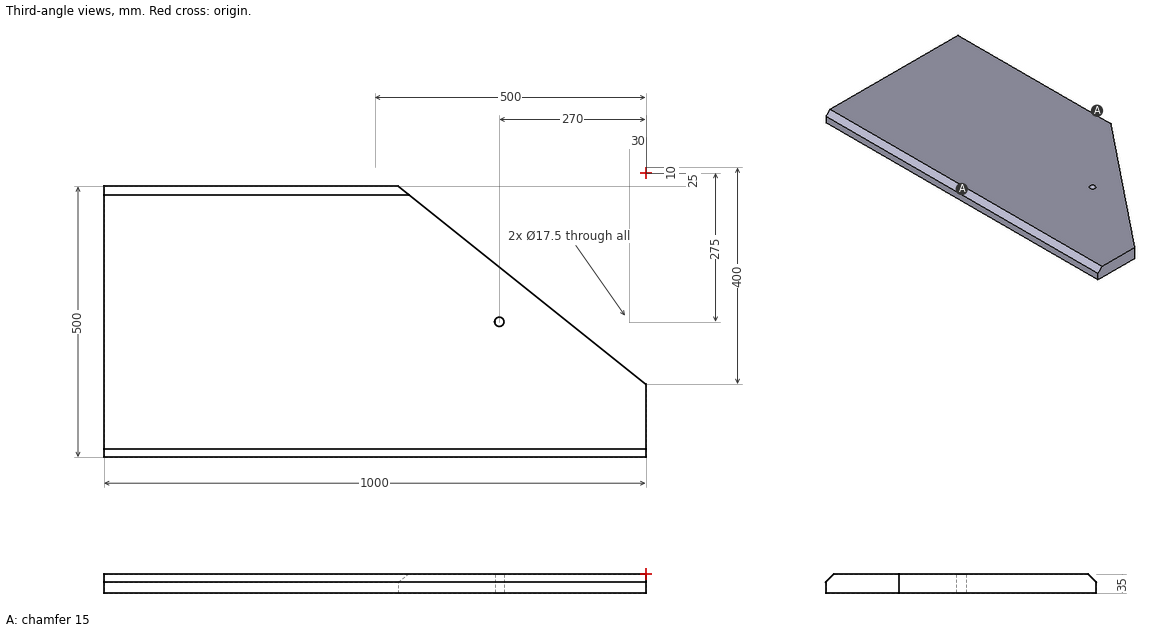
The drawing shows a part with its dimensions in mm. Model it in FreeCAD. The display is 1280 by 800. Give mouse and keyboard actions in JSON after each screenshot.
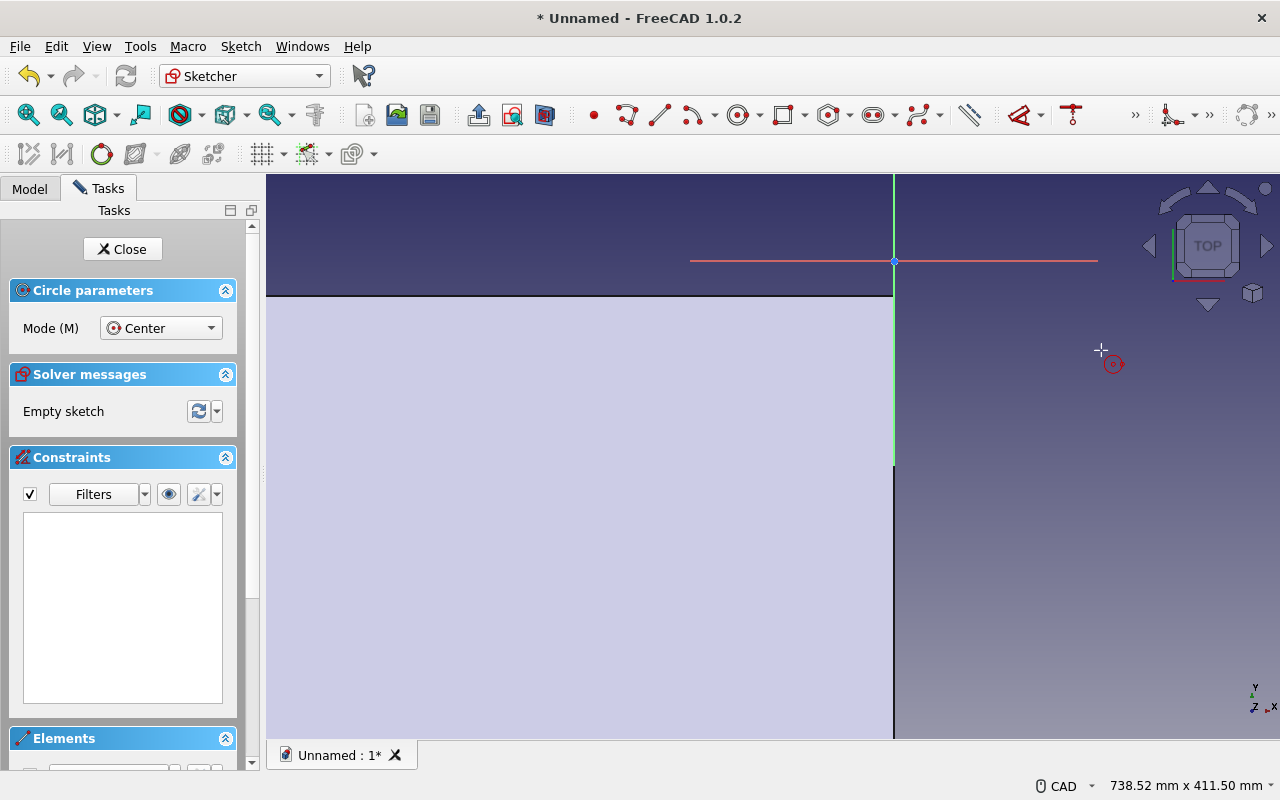
{"action": "scroll", "coordinate": [853, 639], "scroll_direction": "up", "scroll_amount": 4}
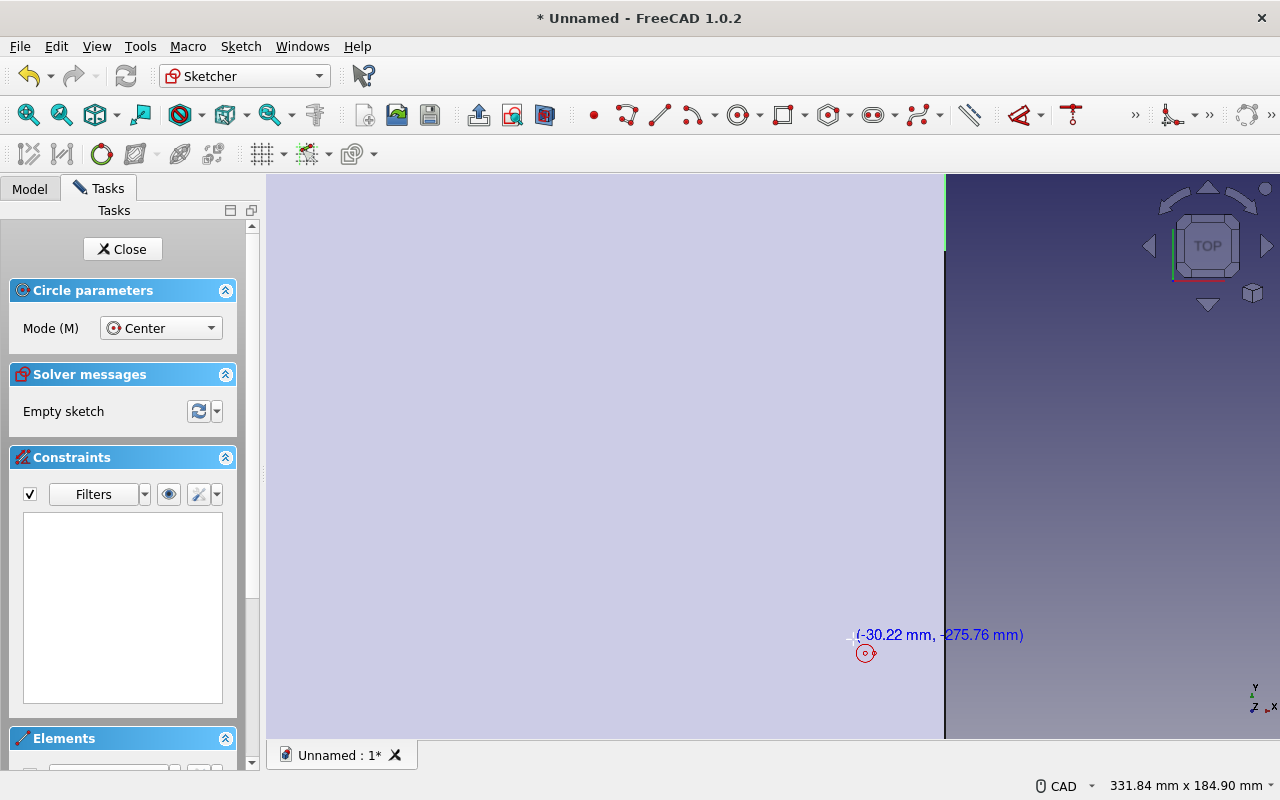
{"action": "left_click", "coordinate": [853, 638]}
{"action": "mouse_move", "coordinate": [872, 619]}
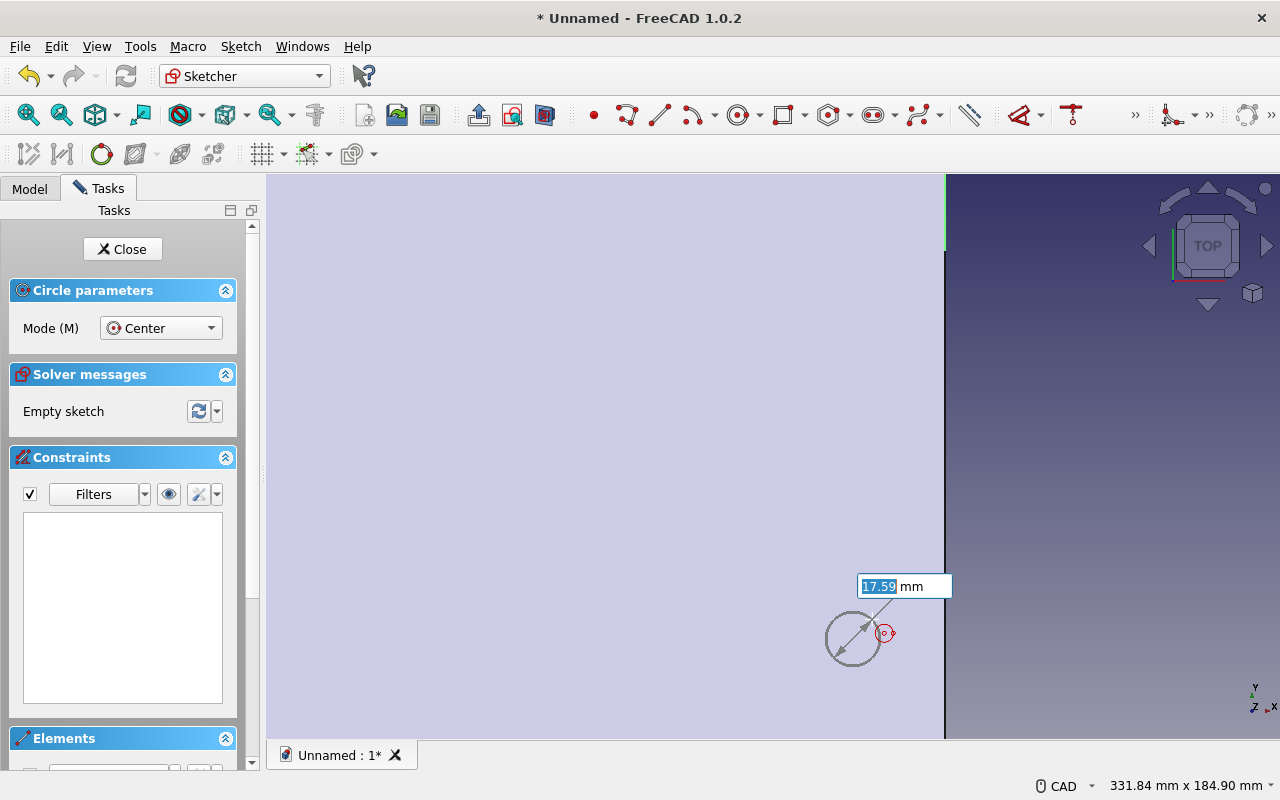
{"action": "type", "text": "17.5"}
{"action": "key", "text": "Return"}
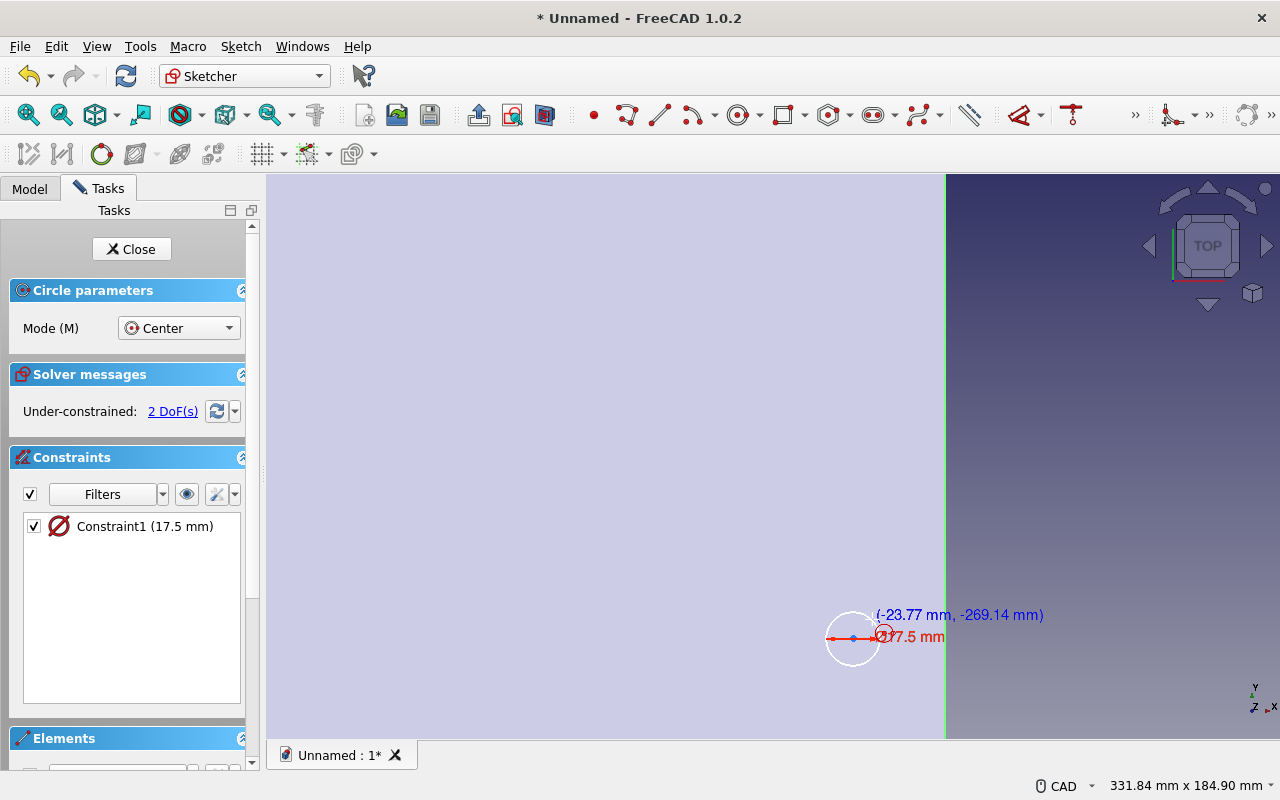
{"action": "scroll", "coordinate": [856, 640], "scroll_direction": "down", "scroll_amount": 4}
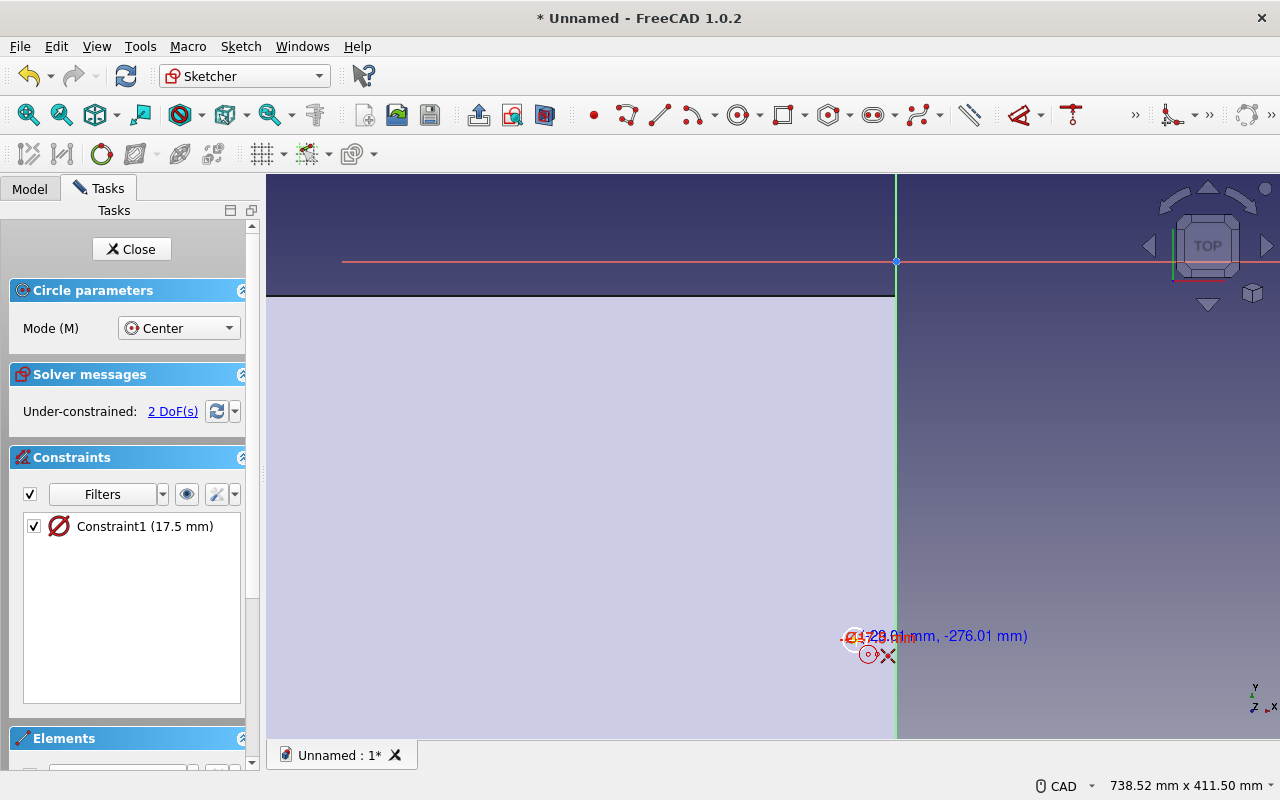
{"action": "scroll", "coordinate": [525, 640], "scroll_direction": "up", "scroll_amount": 4}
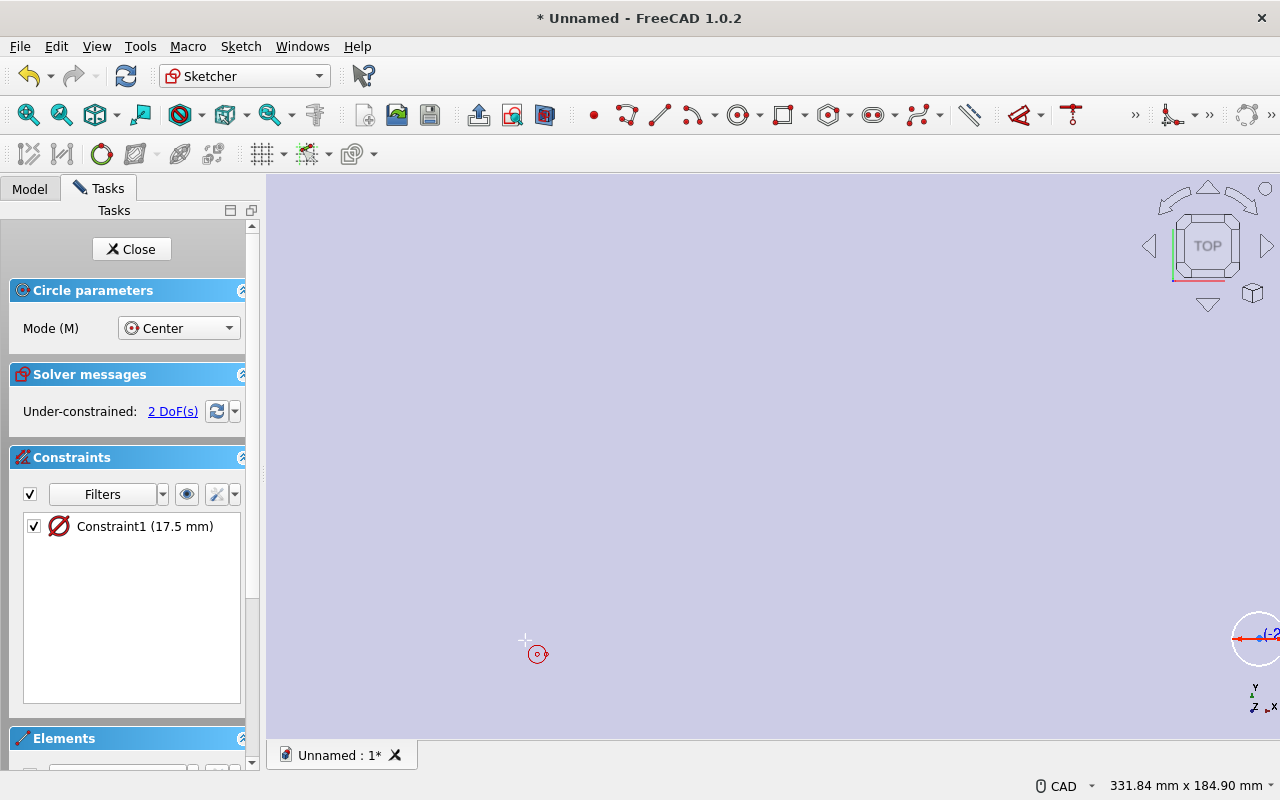
{"action": "left_click", "coordinate": [526, 638]}
{"action": "mouse_move", "coordinate": [545, 619]}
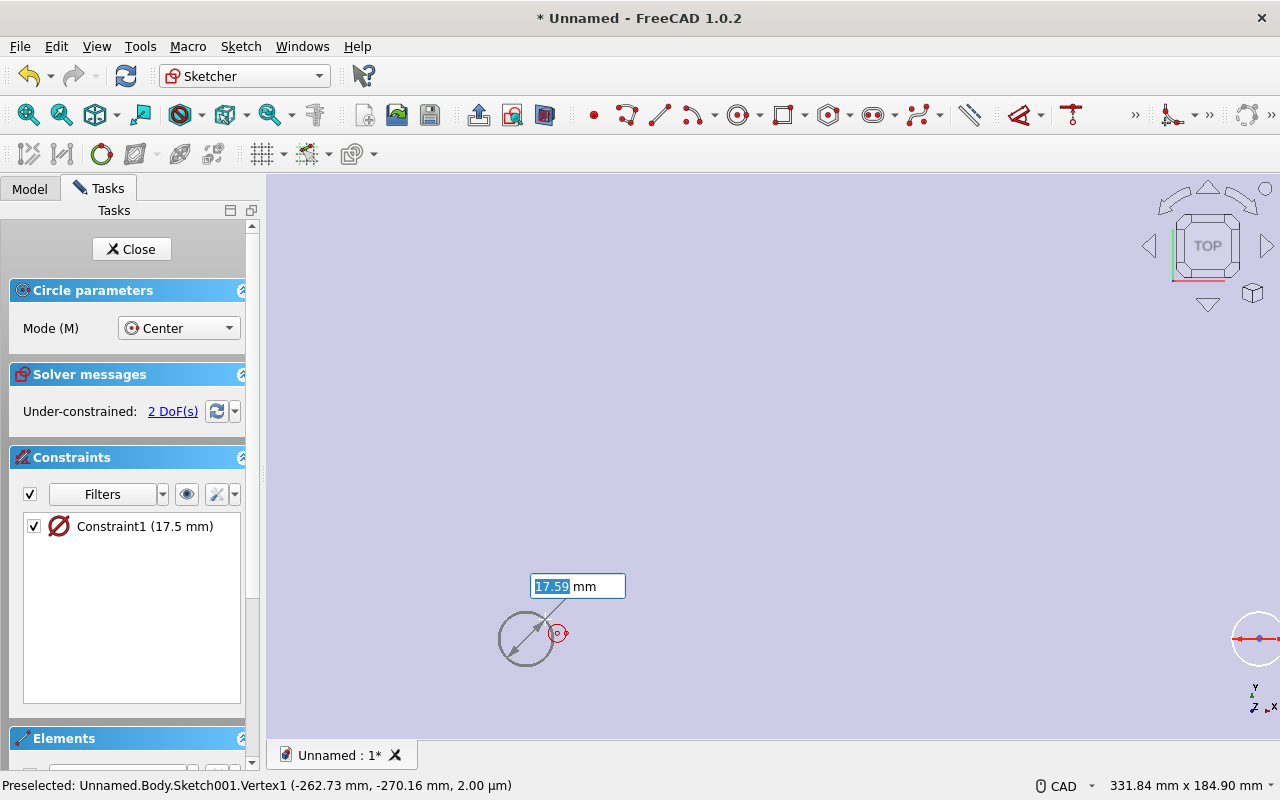
{"action": "type", "text": "17.5"}
{"action": "key", "text": "Return"}
{"action": "key", "text": "Escape"}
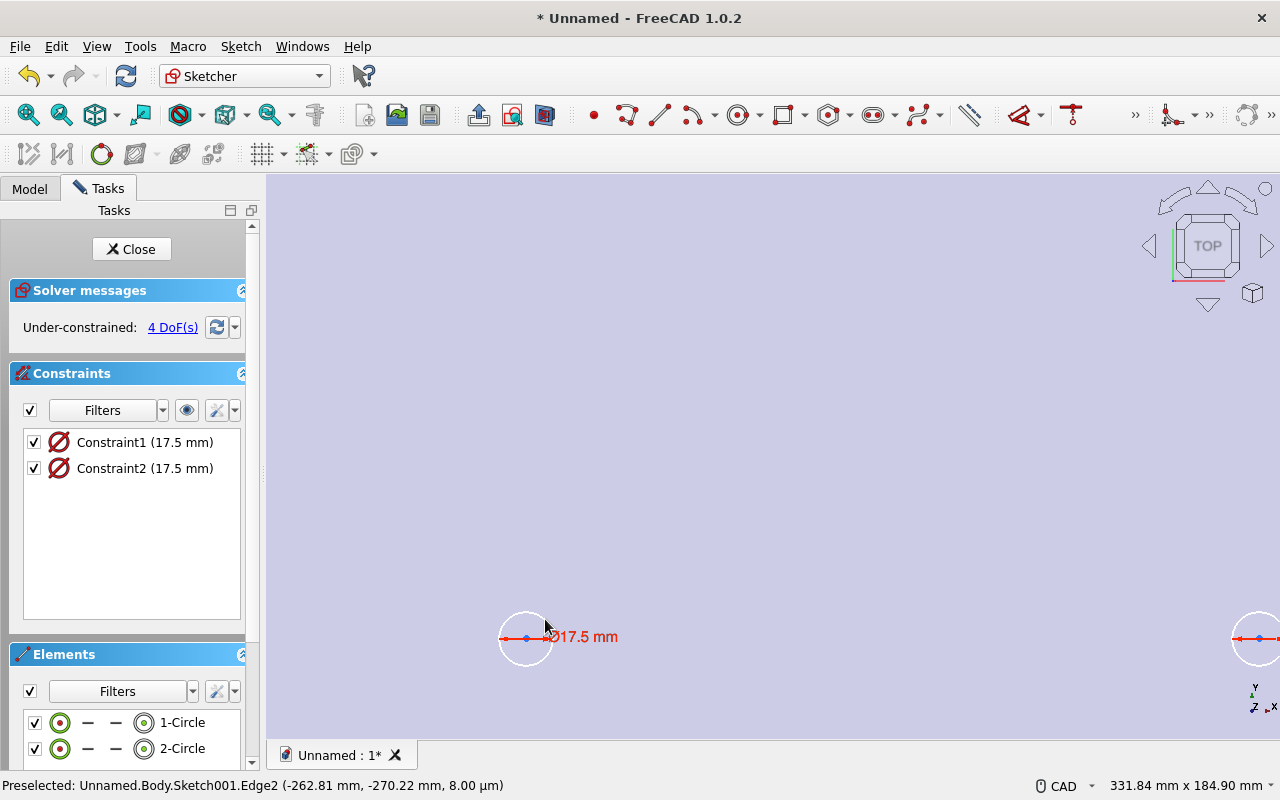
{"action": "scroll", "coordinate": [525, 640], "scroll_direction": "down", "scroll_amount": 4}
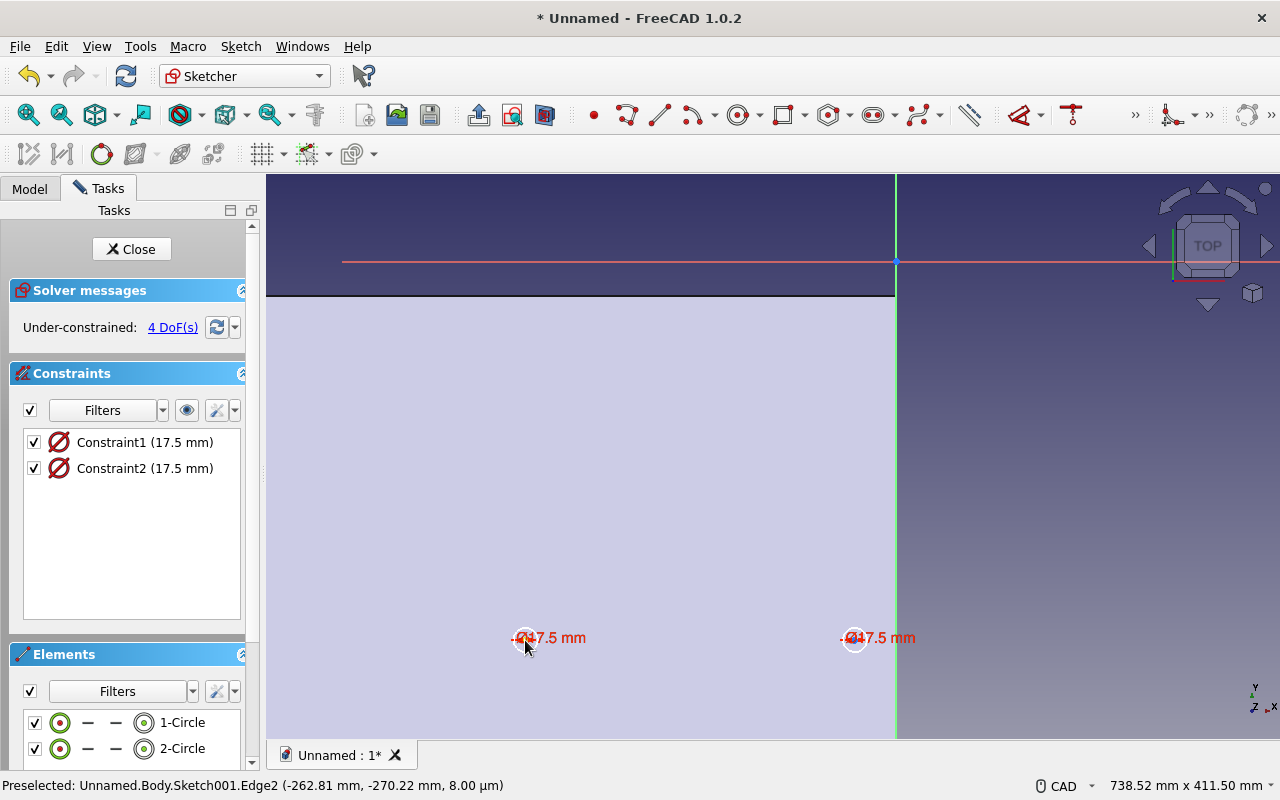
{"action": "left_click", "coordinate": [855, 640]}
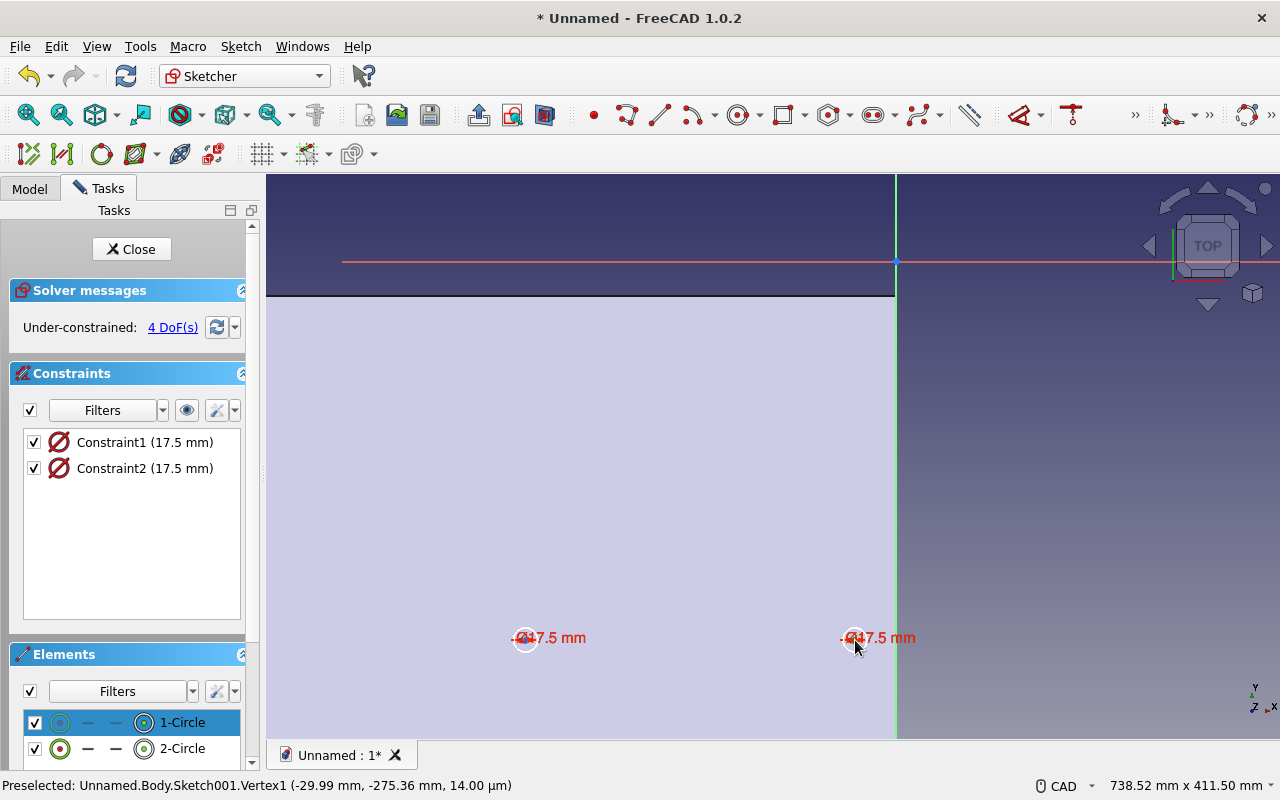
{"action": "left_click", "coordinate": [526, 640]}